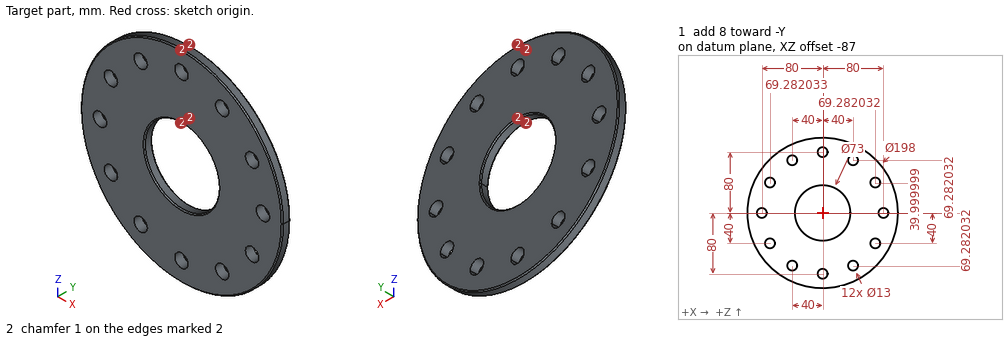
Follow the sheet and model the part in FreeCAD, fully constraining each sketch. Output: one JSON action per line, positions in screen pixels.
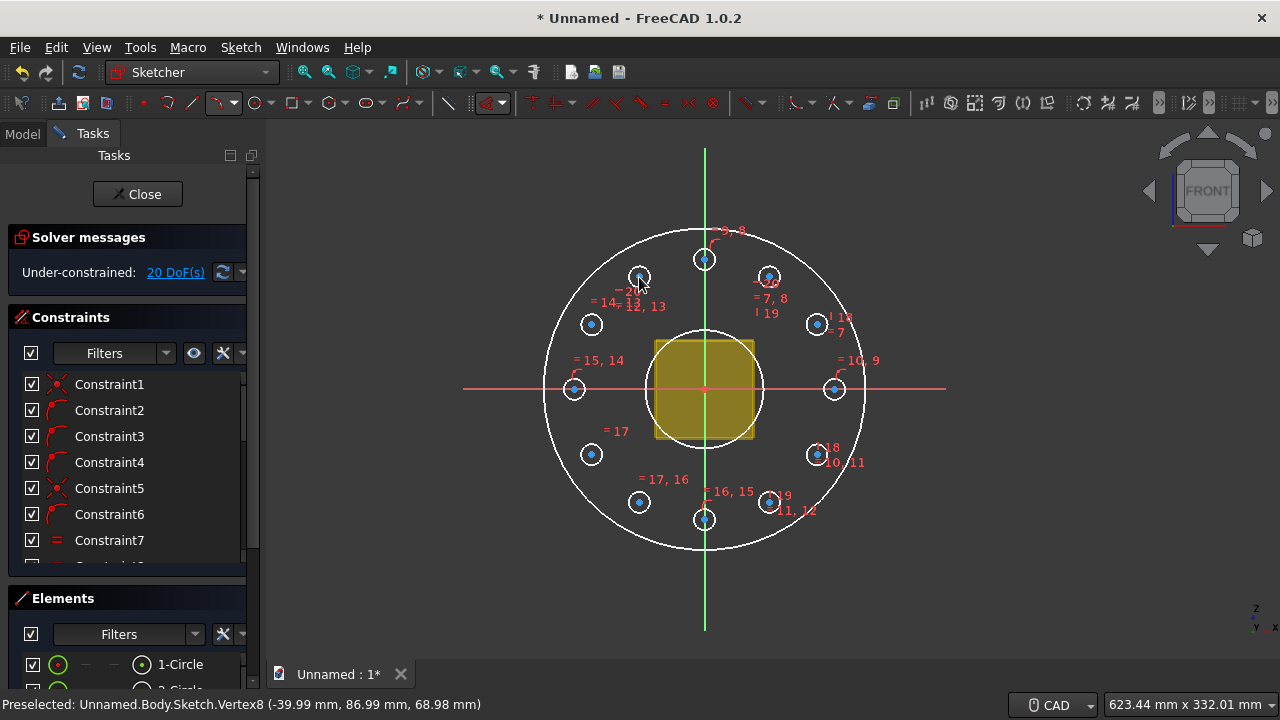
{"action": "left_click", "coordinate": [817, 325]}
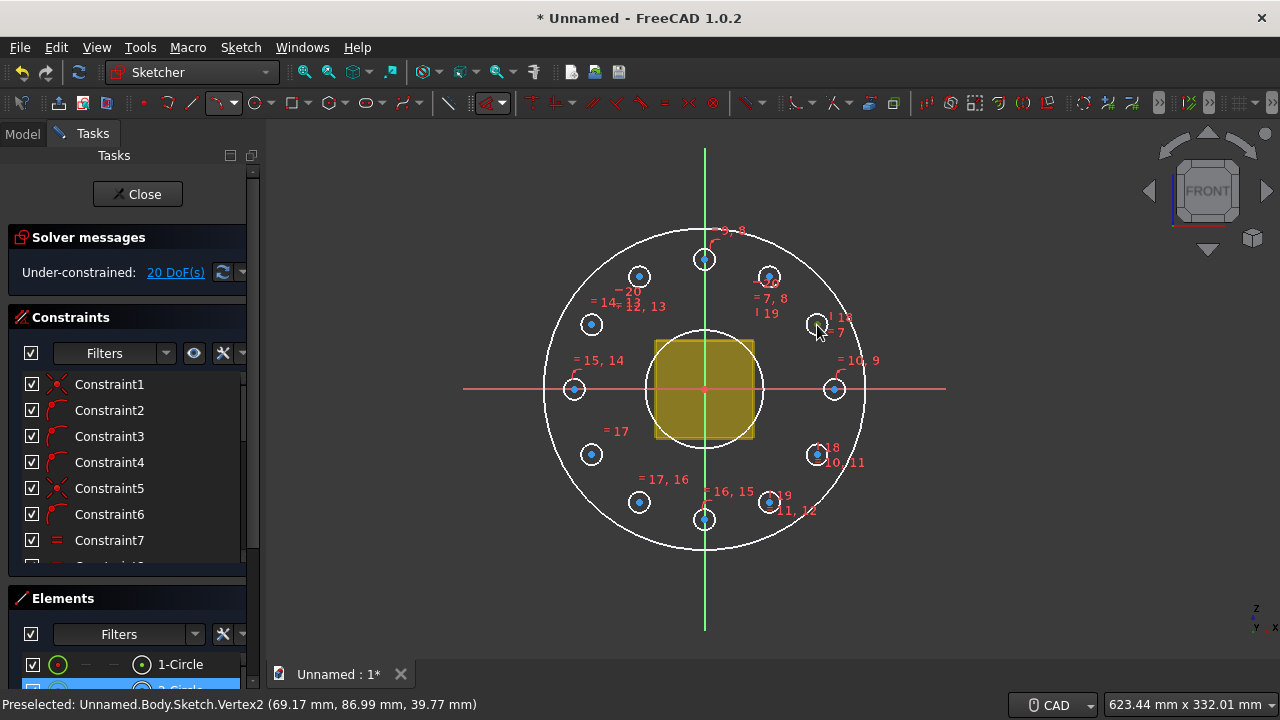
{"action": "left_click", "coordinate": [592, 325]}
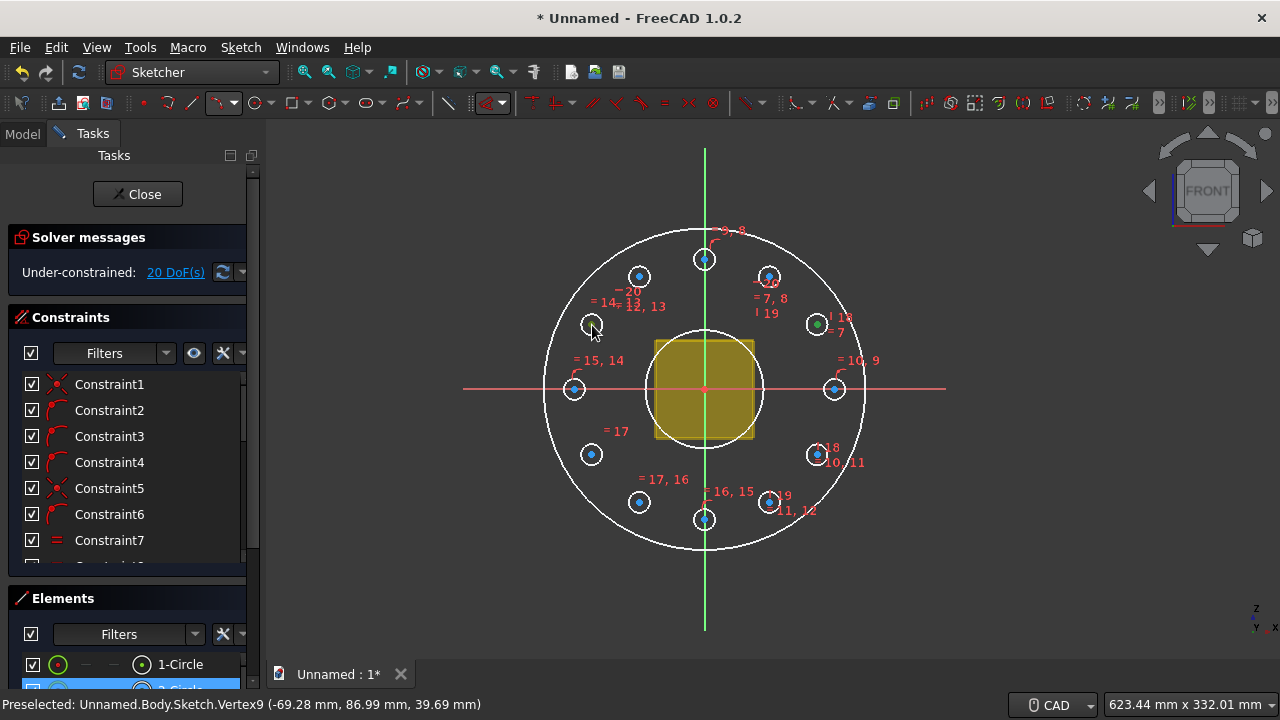
{"action": "left_click", "coordinate": [574, 104]}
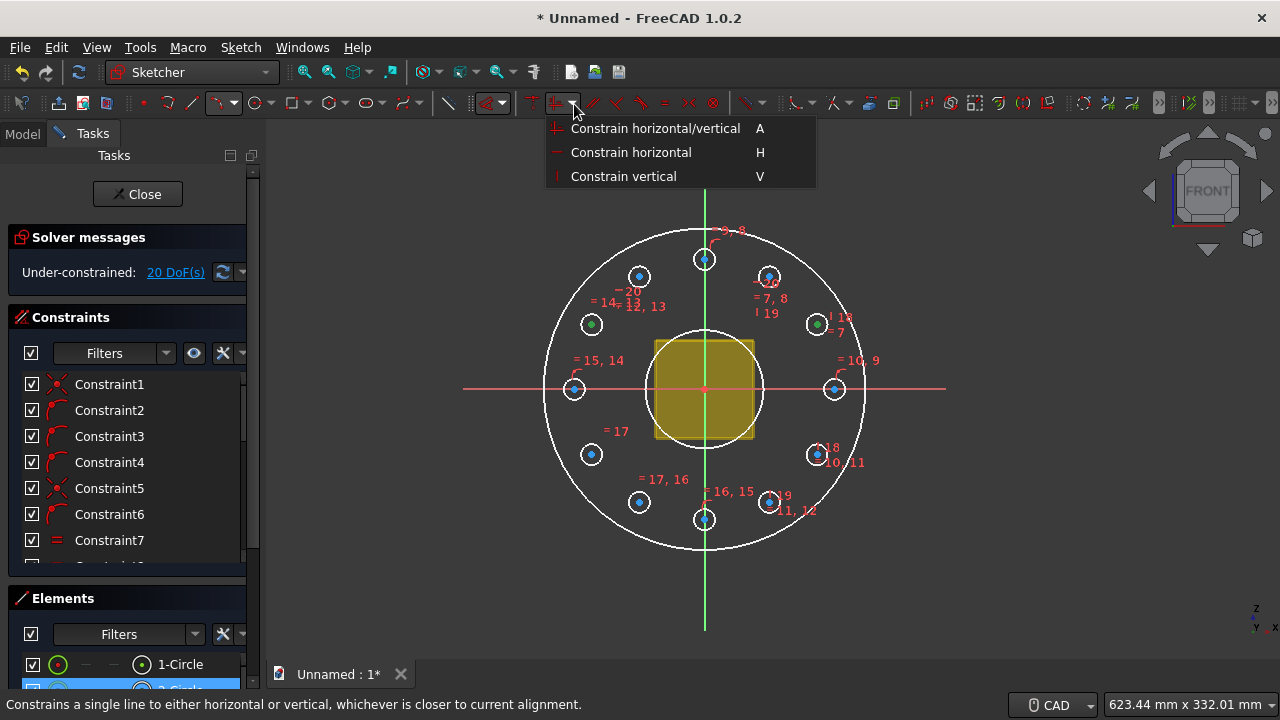
{"action": "left_click", "coordinate": [681, 152]}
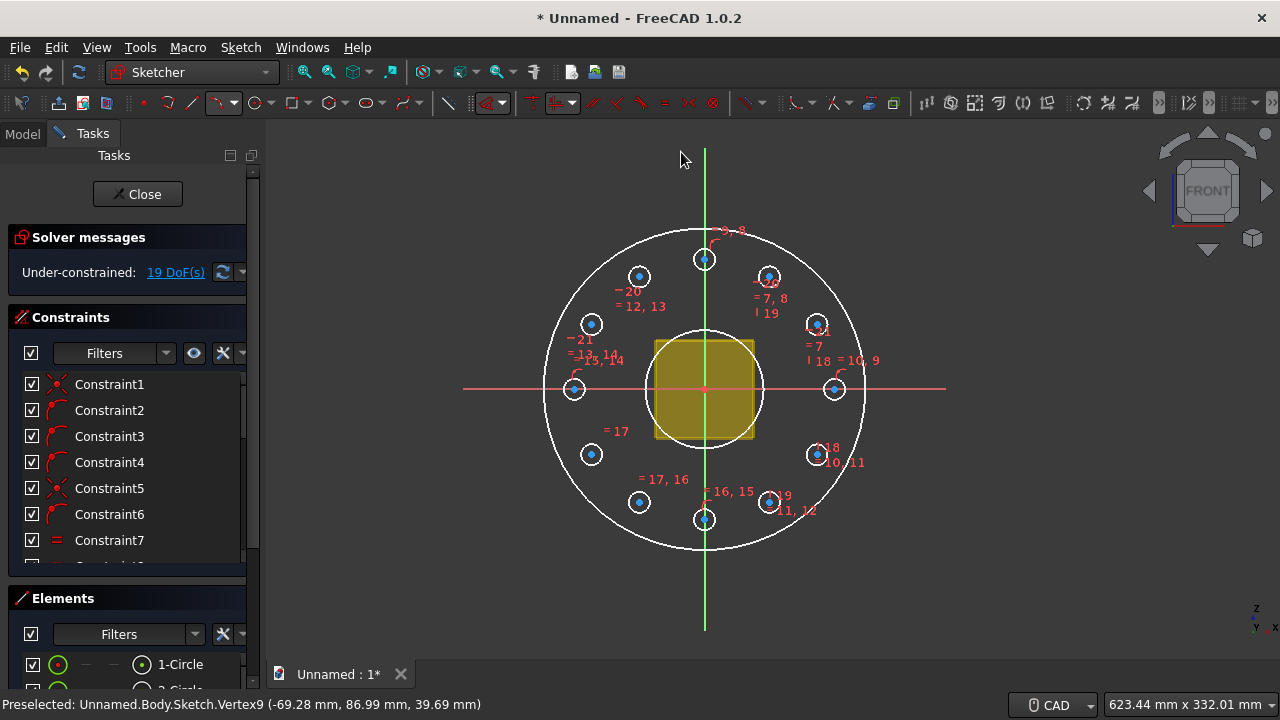
{"action": "scroll", "coordinate": [769, 502], "scroll_direction": "up", "scroll_amount": 4}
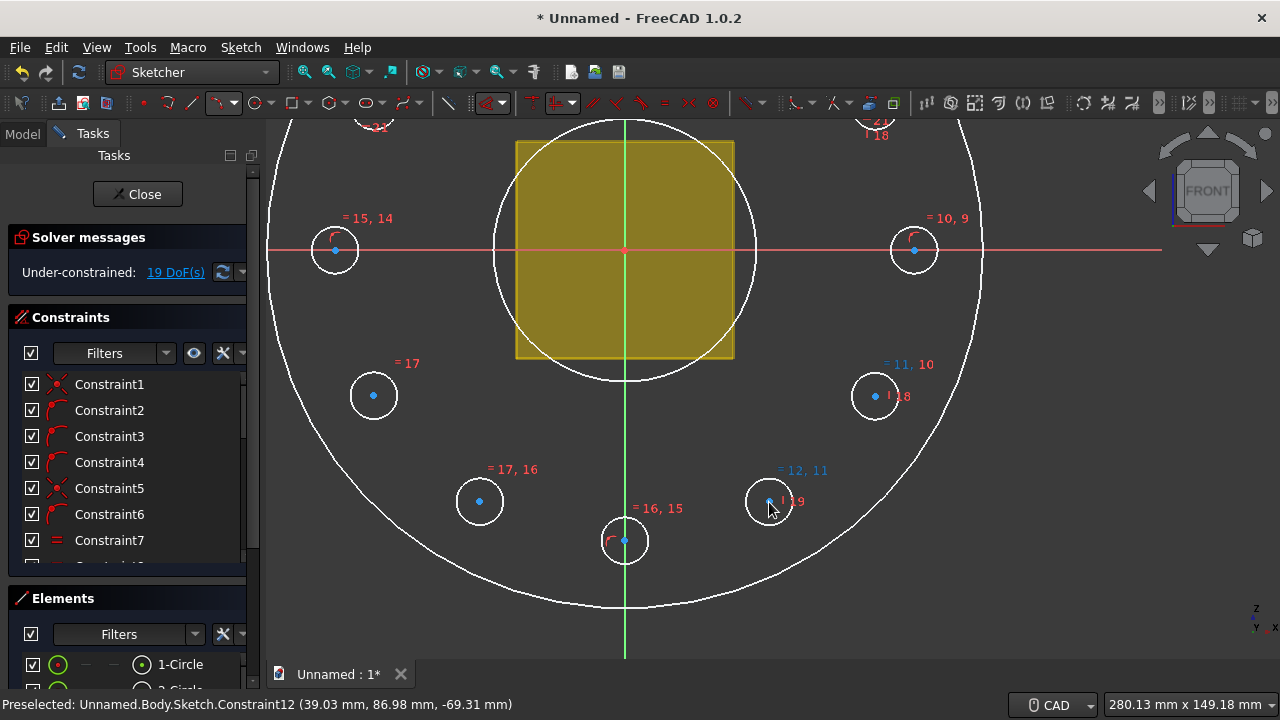
{"action": "left_click", "coordinate": [769, 502]}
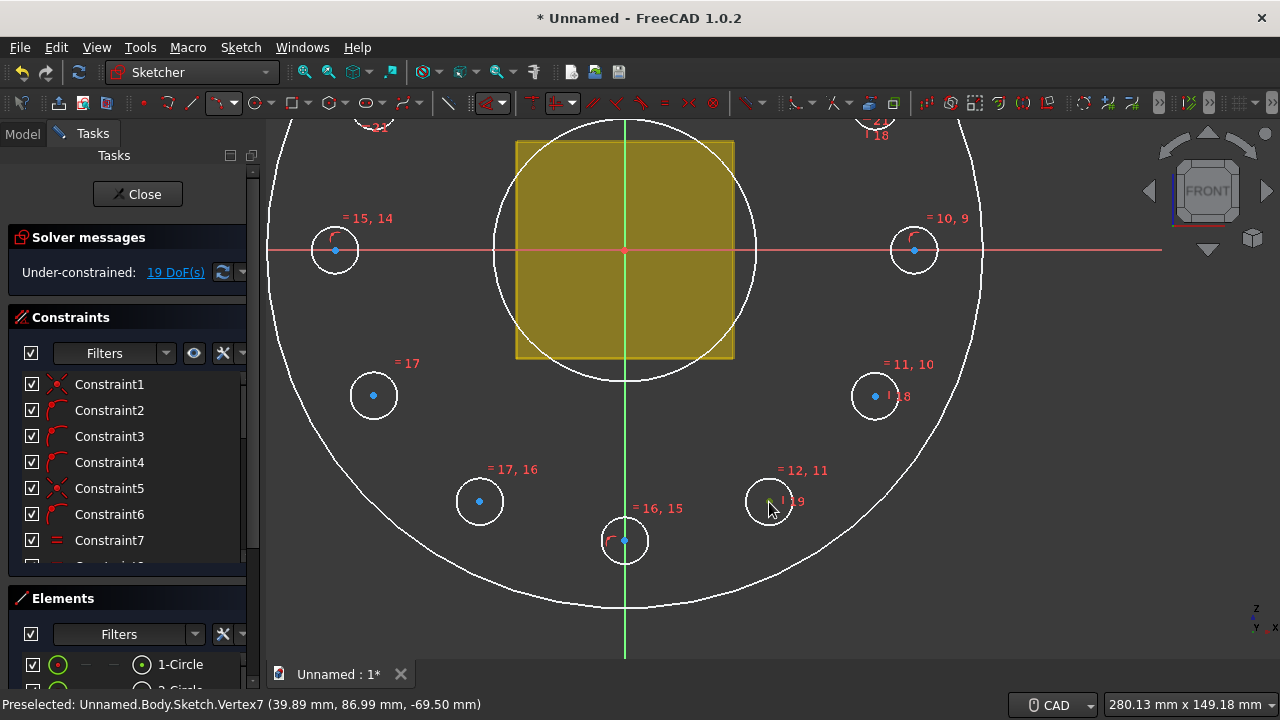
{"action": "left_click", "coordinate": [480, 502]}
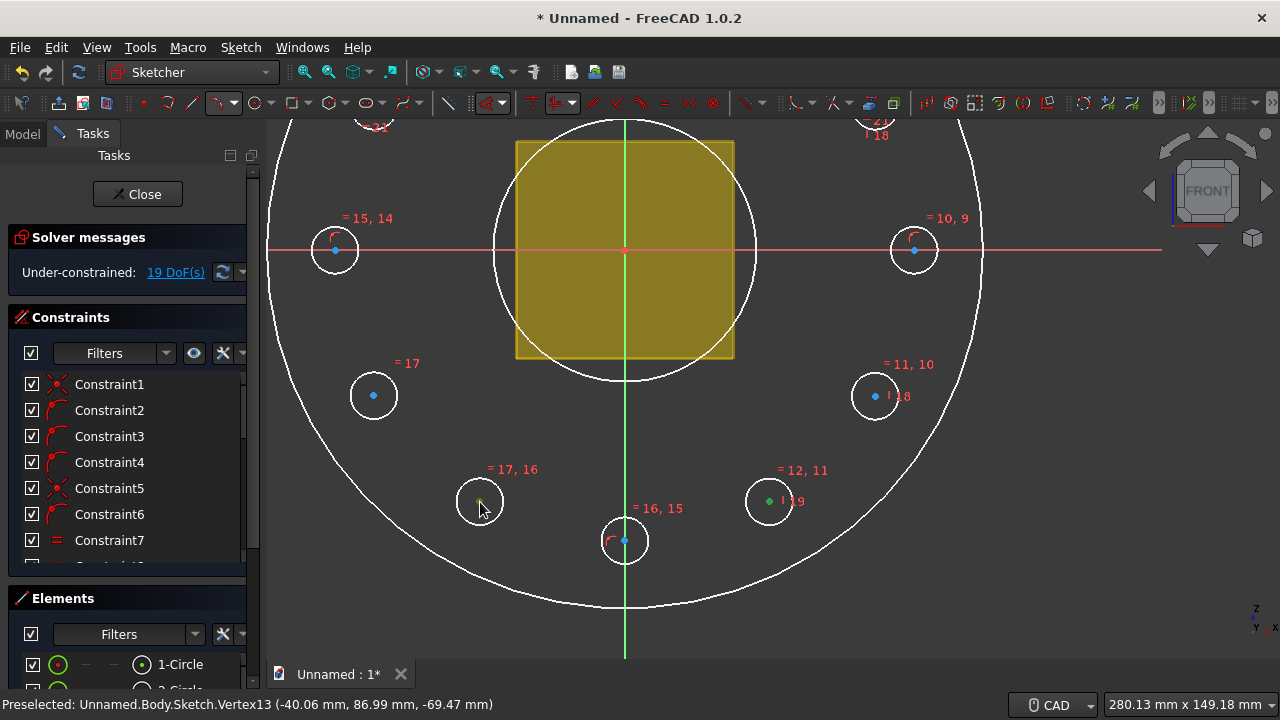
{"action": "key", "text": "h"}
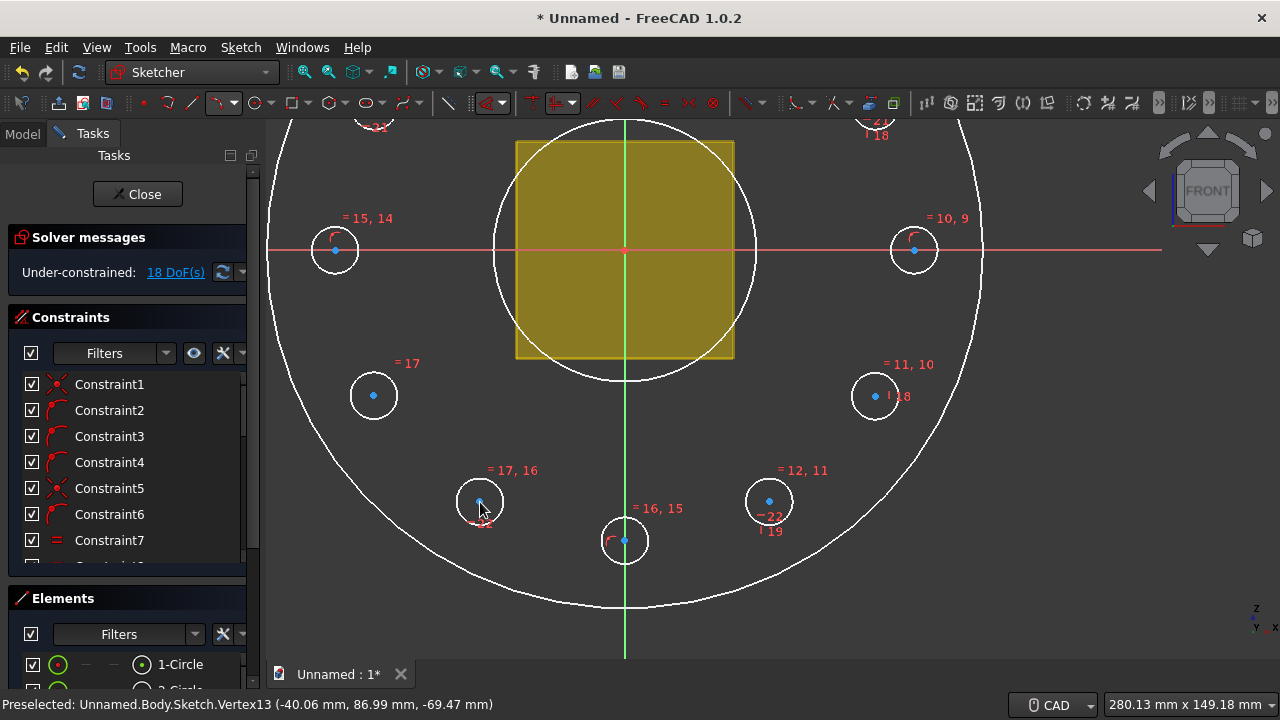
{"action": "scroll", "coordinate": [769, 502], "scroll_direction": "down", "scroll_amount": 4}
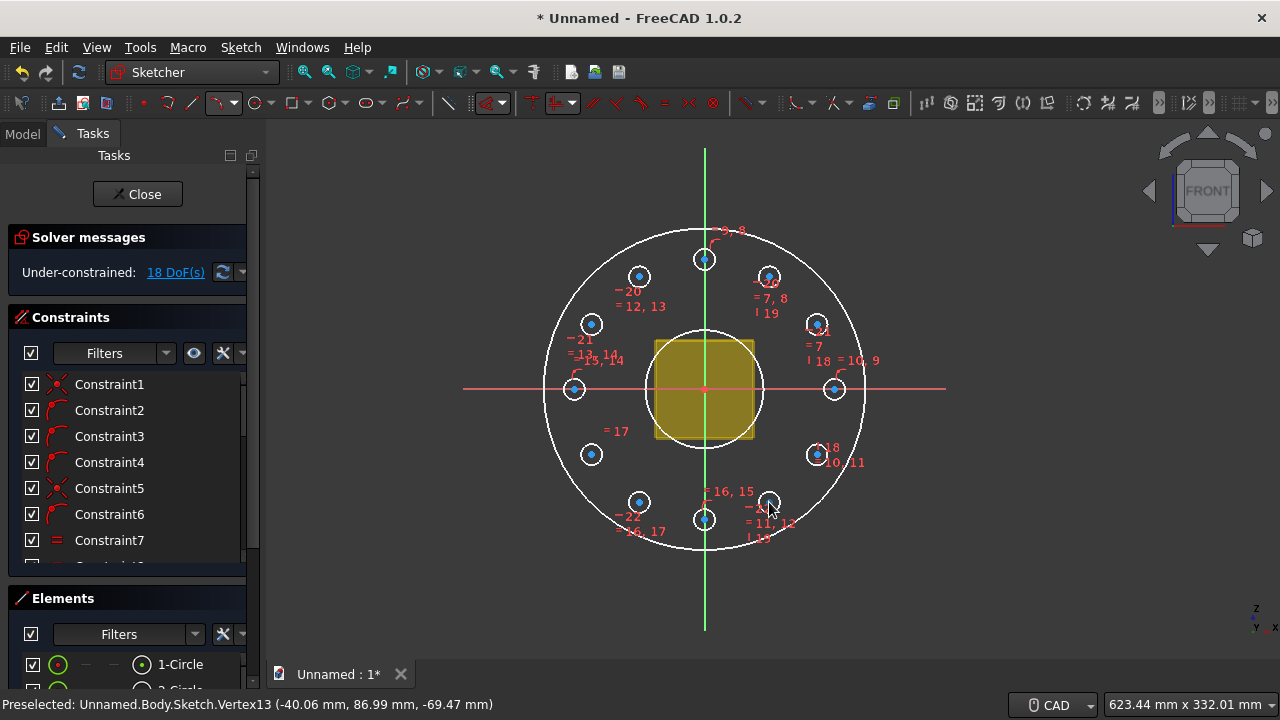
{"action": "left_click", "coordinate": [592, 325]}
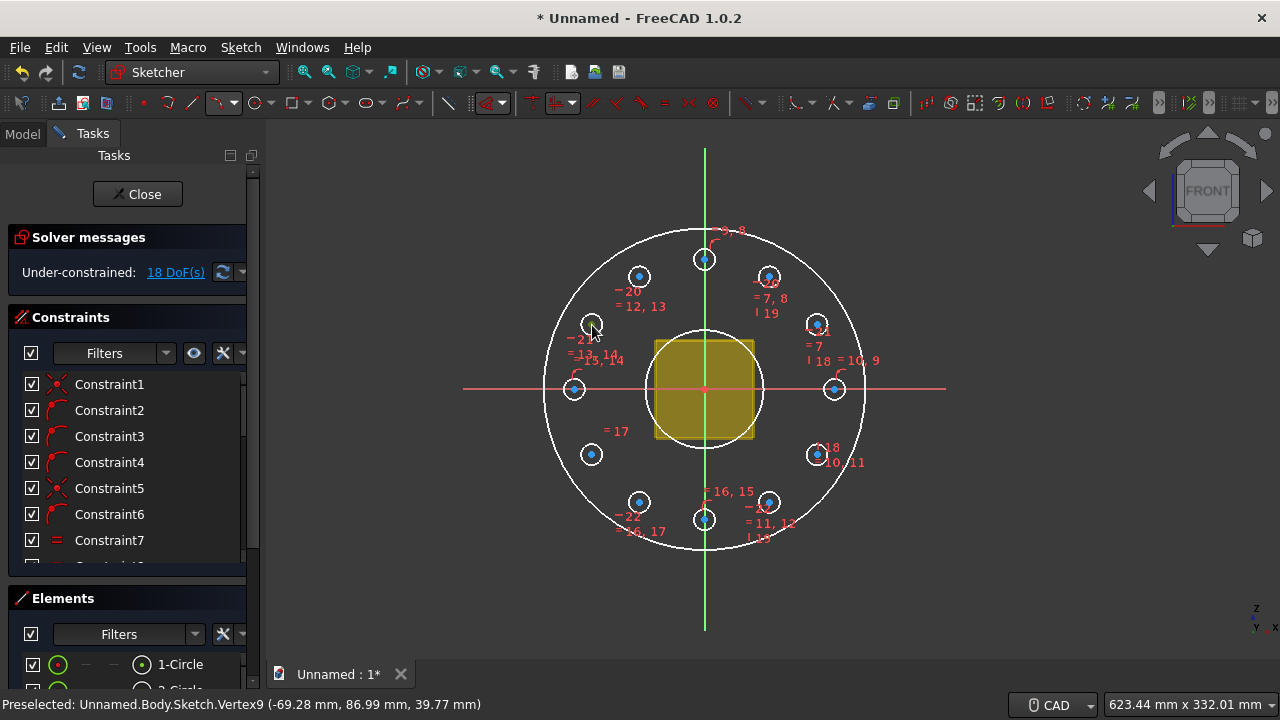
{"action": "left_click", "coordinate": [592, 455]}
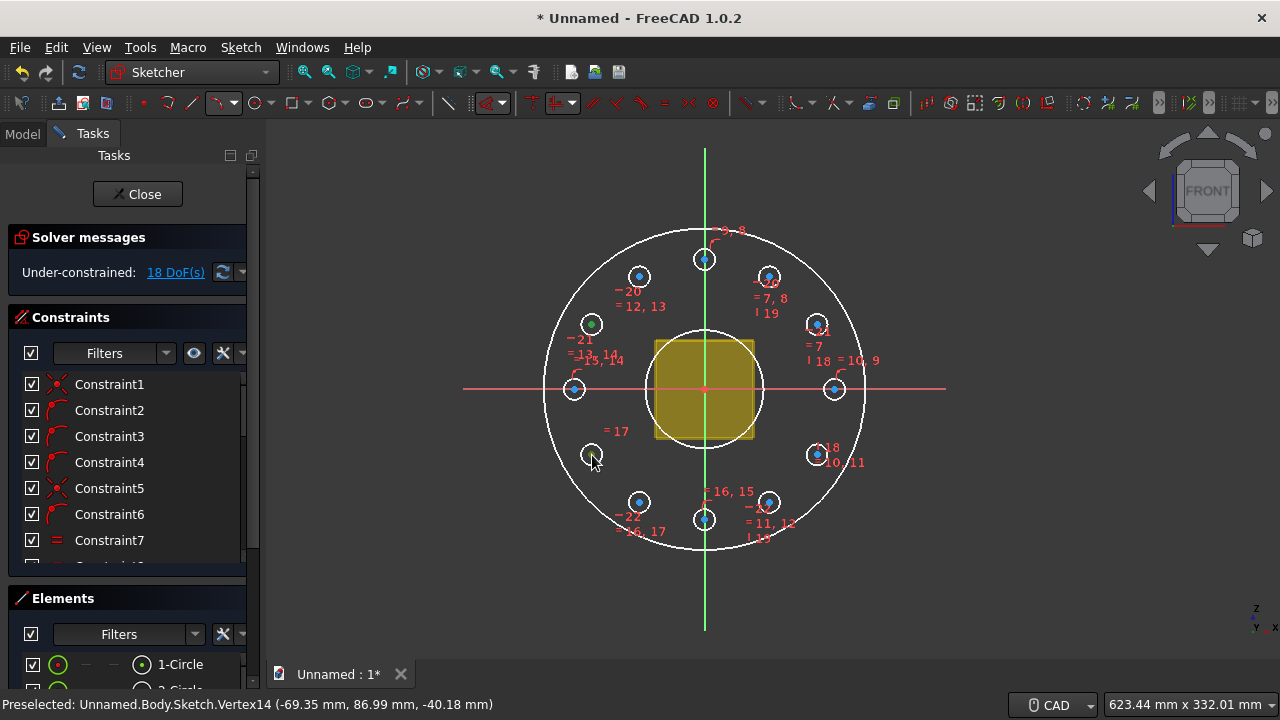
{"action": "key", "text": "v"}